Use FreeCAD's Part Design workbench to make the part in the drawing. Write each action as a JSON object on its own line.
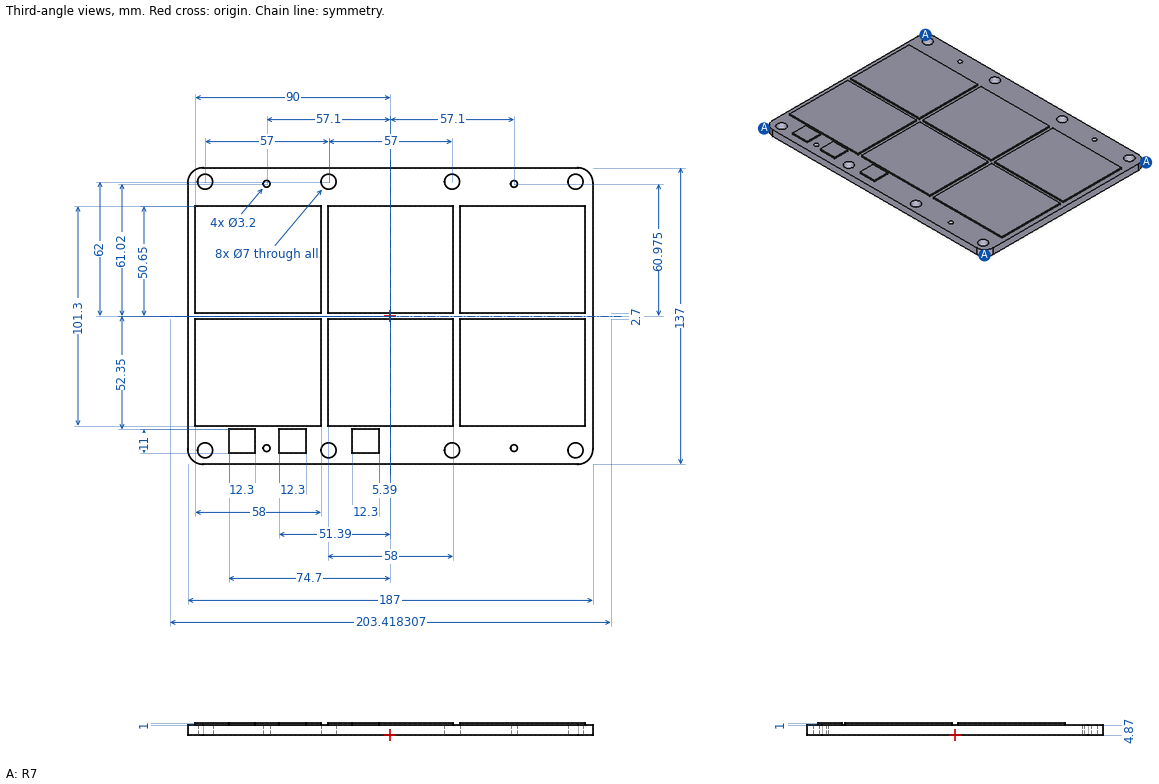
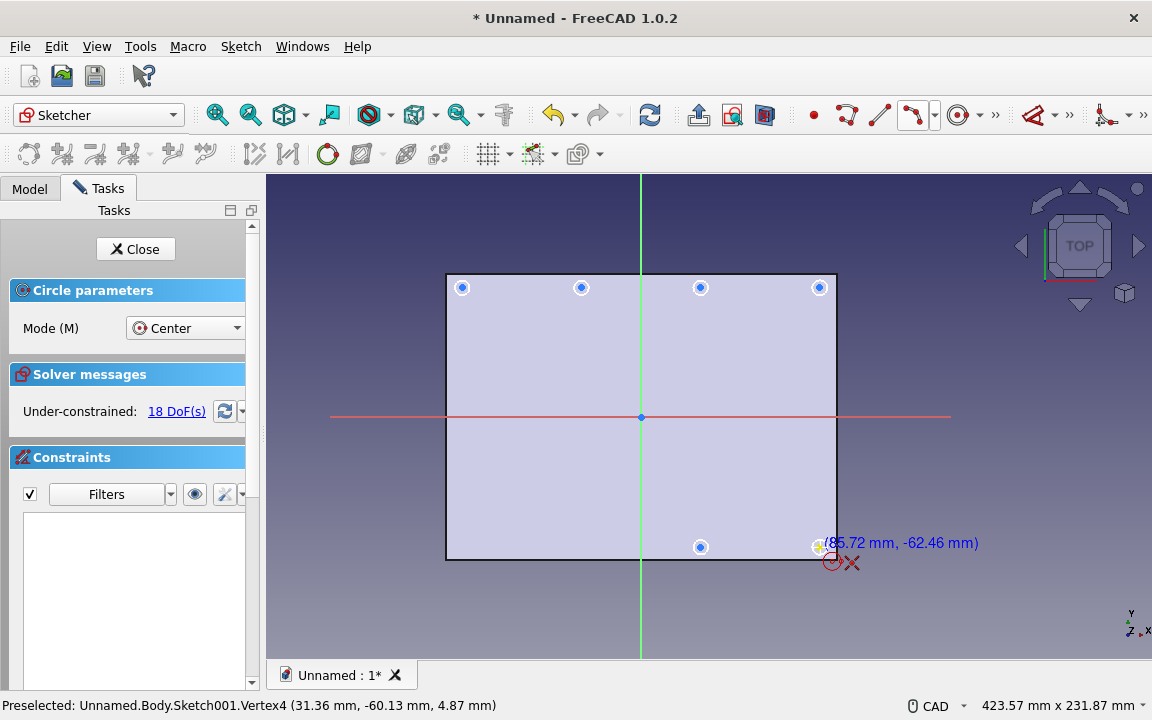
{"action": "scroll", "coordinate": [462, 547], "scroll_direction": "up", "scroll_amount": 6}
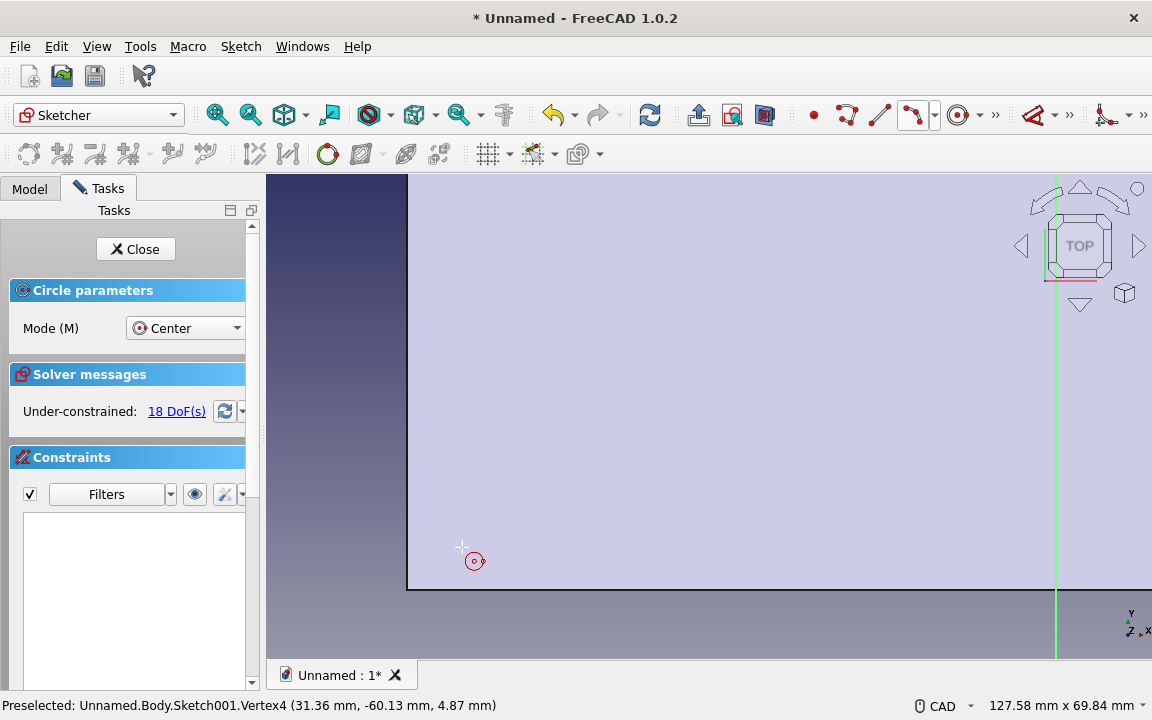
{"action": "left_click", "coordinate": [462, 545]}
{"action": "left_click", "coordinate": [480, 528]}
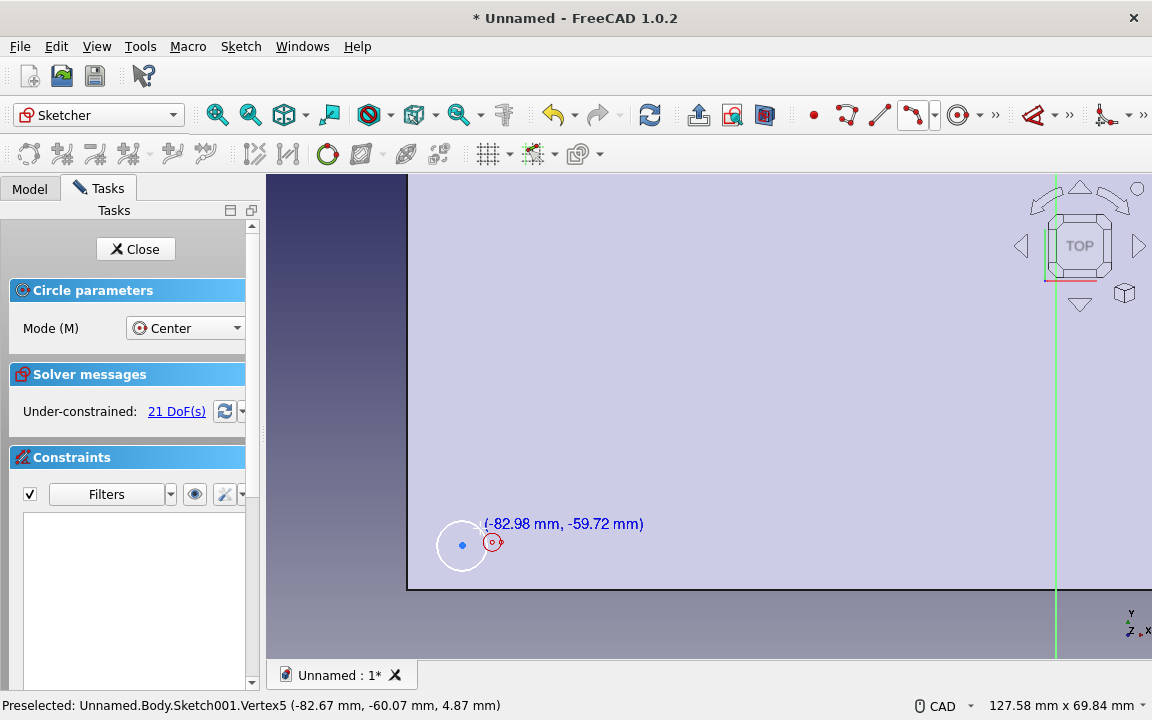
{"action": "left_click", "coordinate": [858, 545]}
{"action": "left_click", "coordinate": [876, 528]}
{"action": "key", "text": "Escape"}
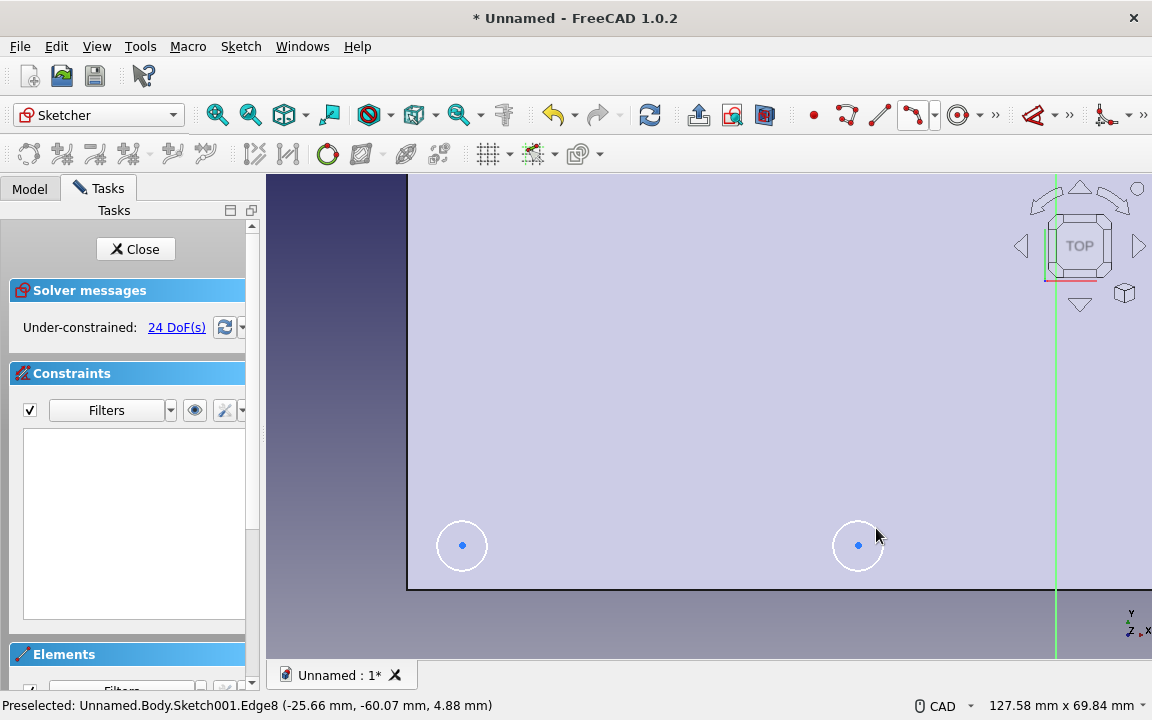
{"action": "scroll", "coordinate": [461, 547], "scroll_direction": "down", "scroll_amount": 6}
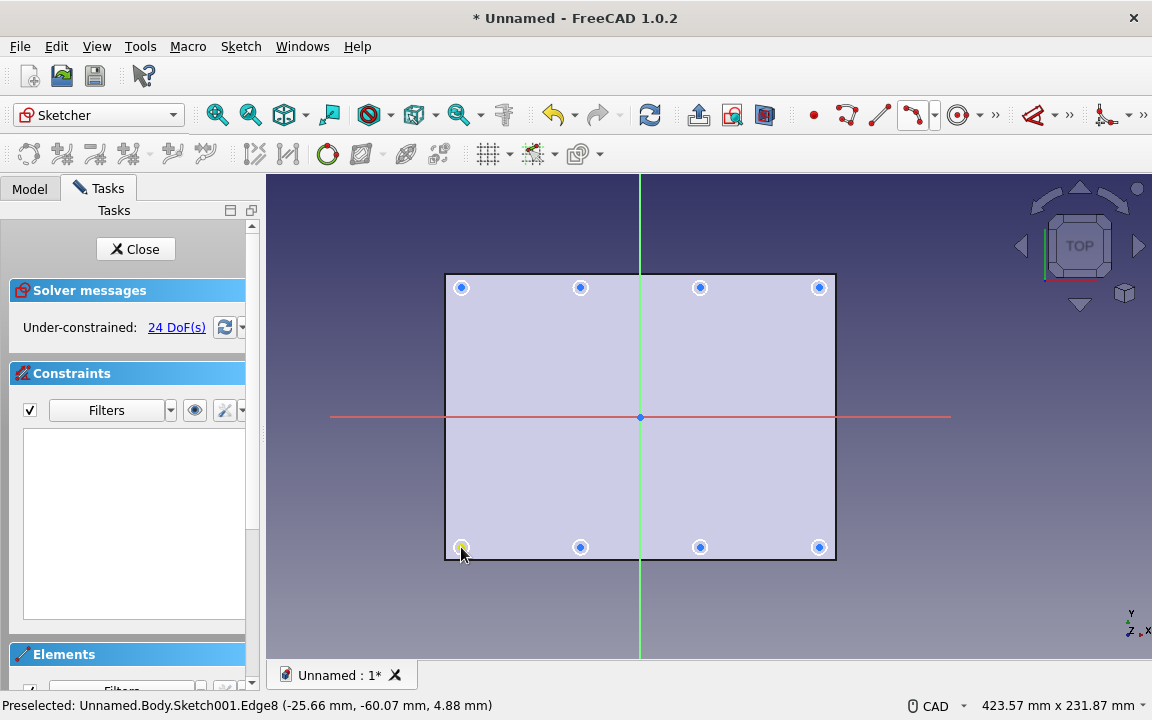
{"action": "scroll", "coordinate": [586, 283], "scroll_direction": "up", "scroll_amount": 4}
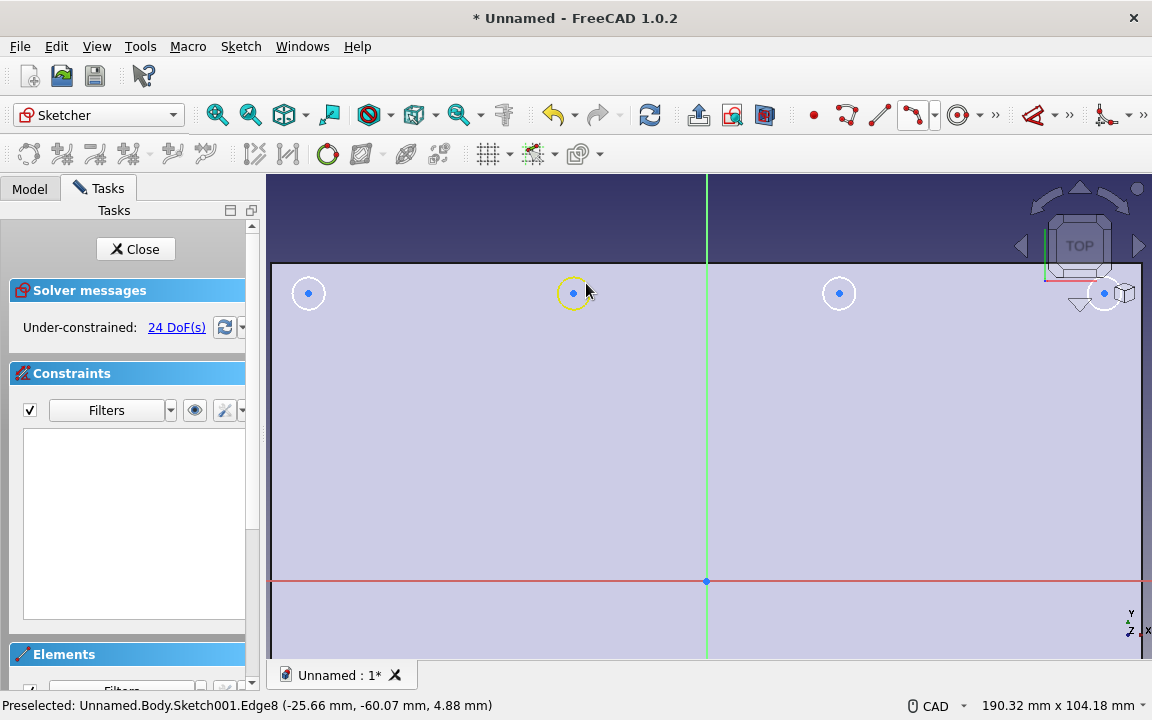
{"action": "left_click", "coordinate": [585, 282]}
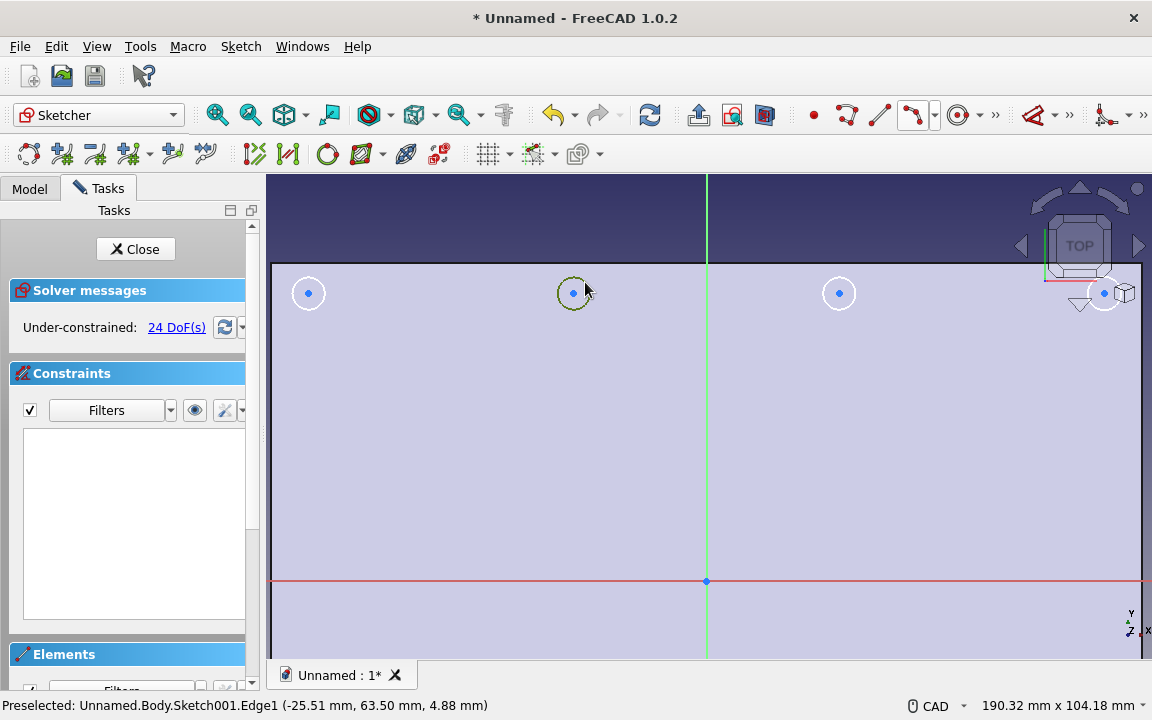
{"action": "left_click", "coordinate": [320, 282]}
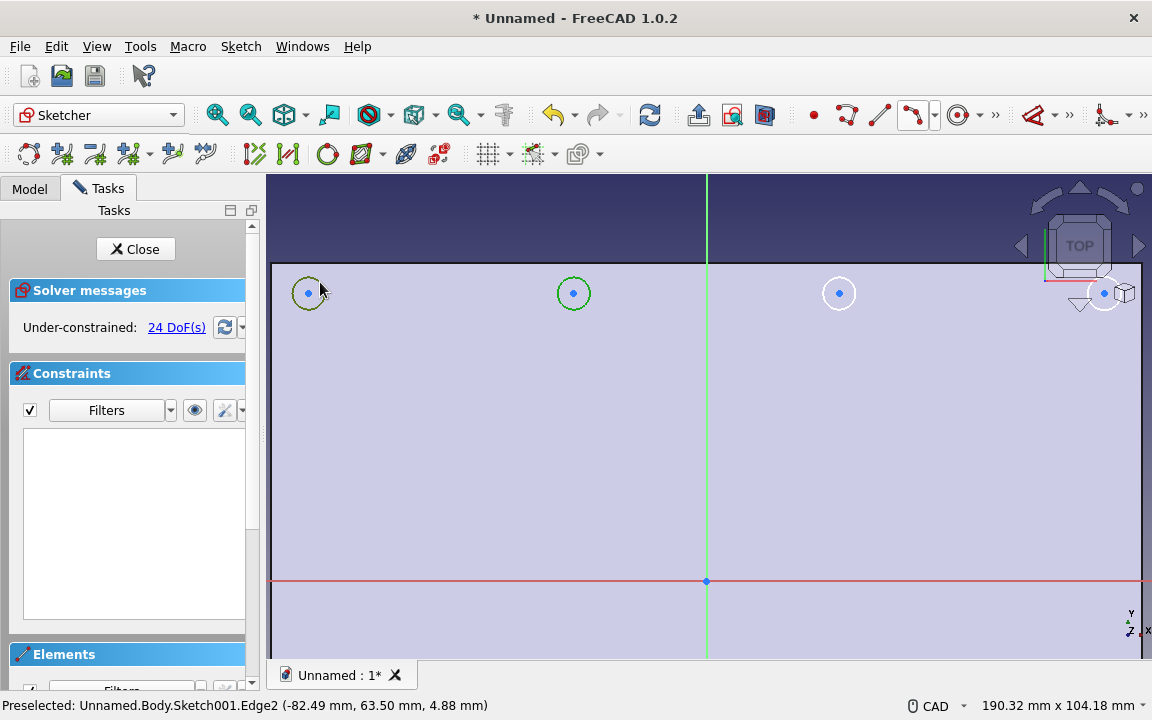
{"action": "left_click", "coordinate": [851, 282]}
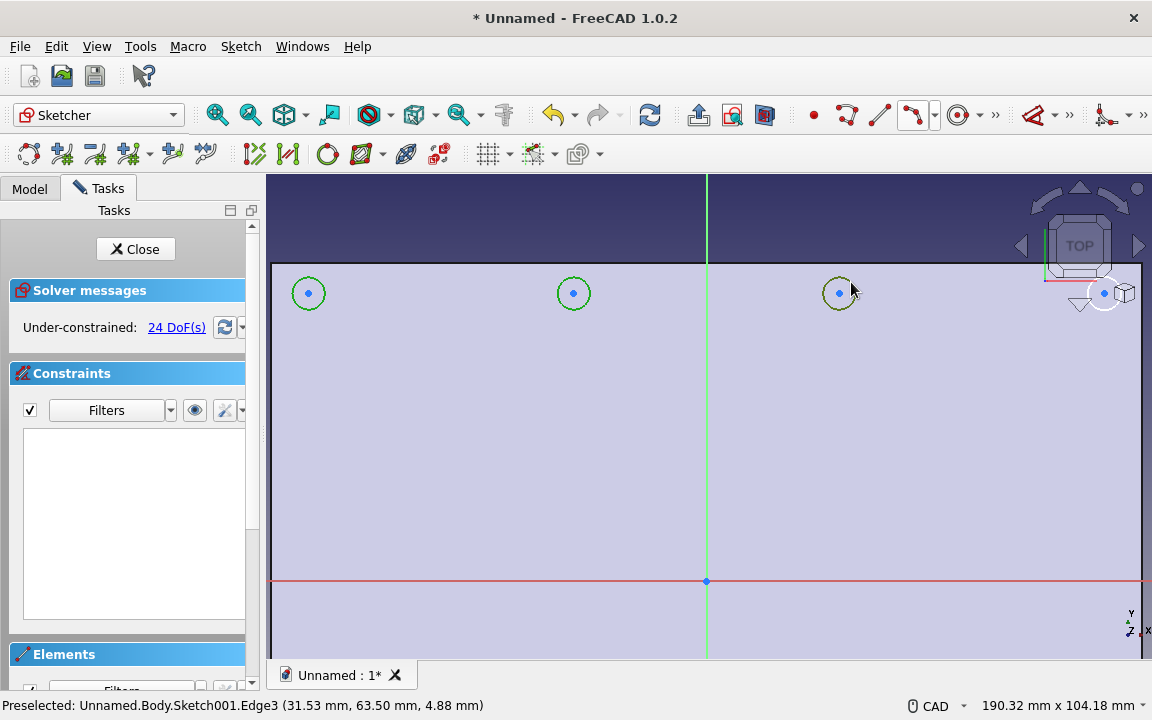
{"action": "scroll", "coordinate": [586, 282], "scroll_direction": "down", "scroll_amount": 4}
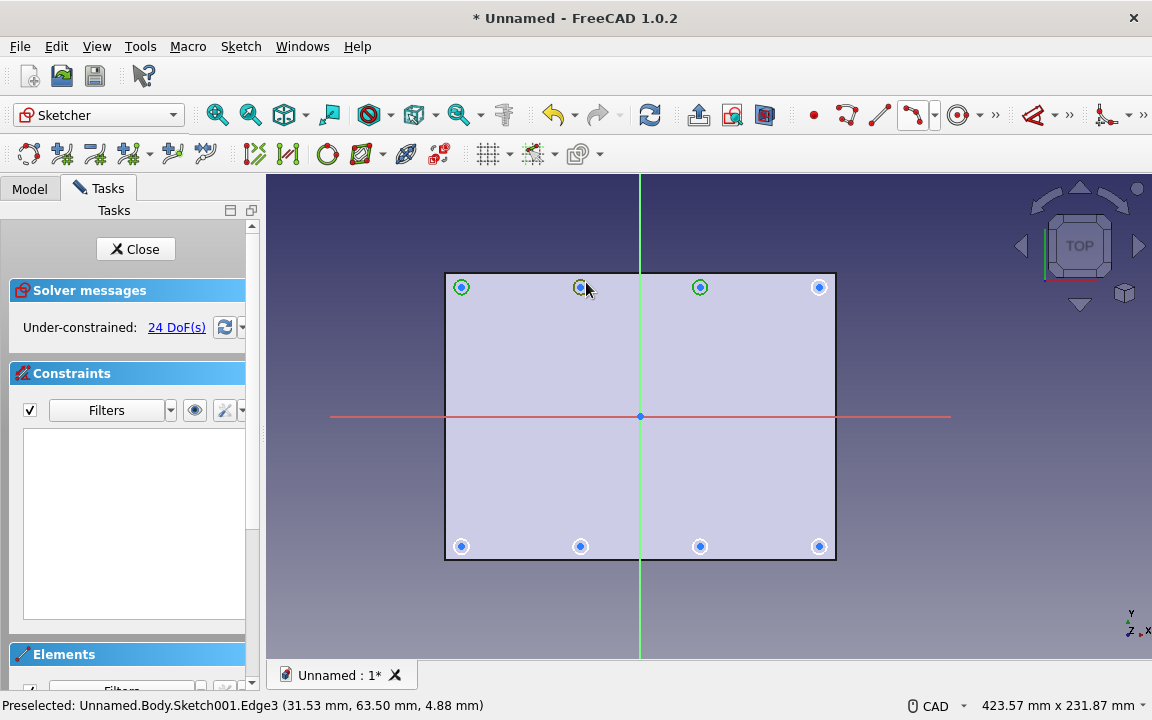
{"action": "scroll", "coordinate": [824, 282], "scroll_direction": "up", "scroll_amount": 4}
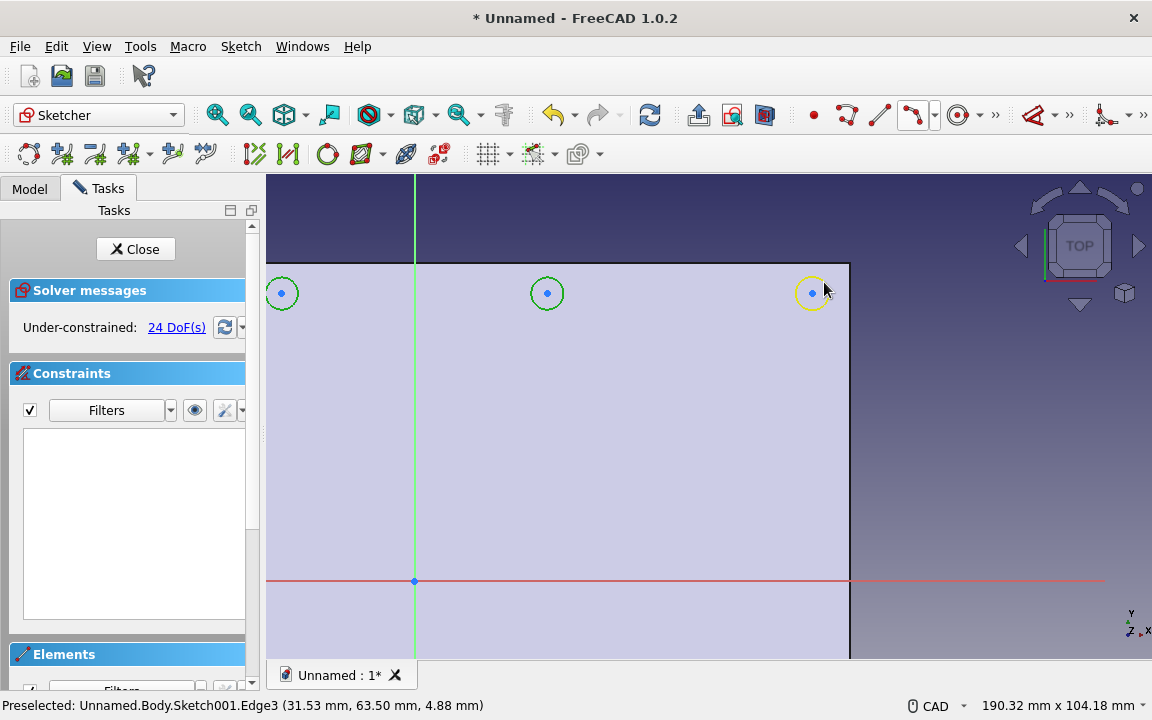
{"action": "left_click", "coordinate": [824, 282]}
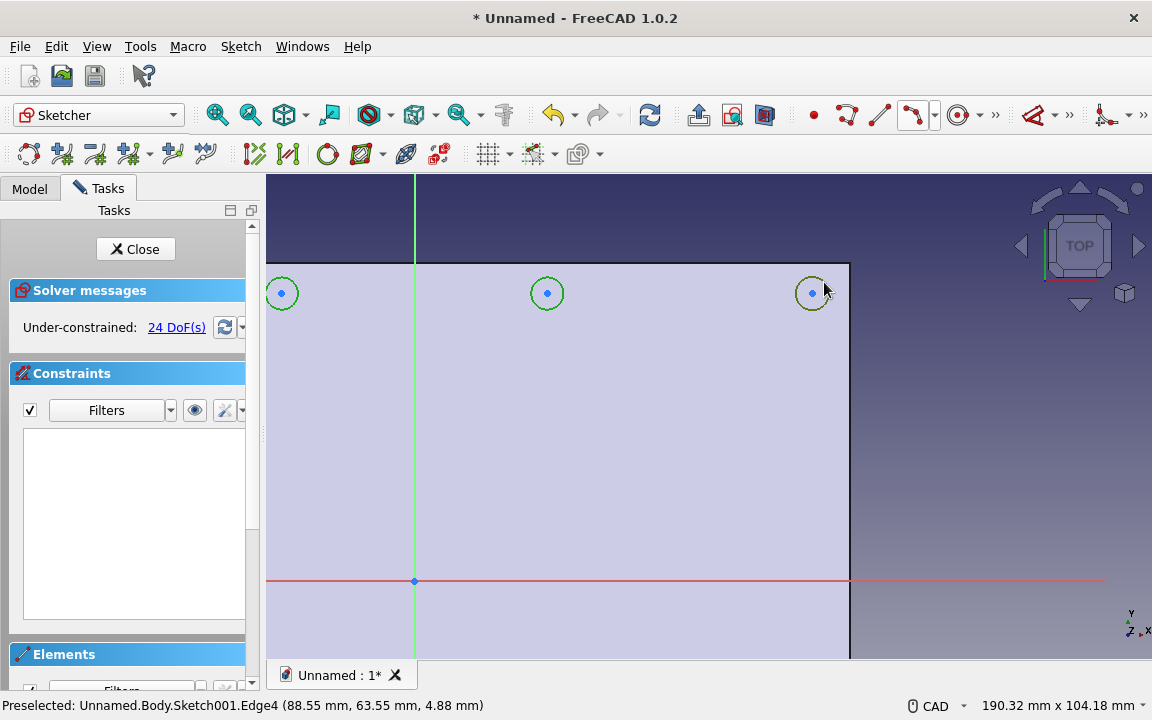
{"action": "scroll", "coordinate": [825, 282], "scroll_direction": "down", "scroll_amount": 4}